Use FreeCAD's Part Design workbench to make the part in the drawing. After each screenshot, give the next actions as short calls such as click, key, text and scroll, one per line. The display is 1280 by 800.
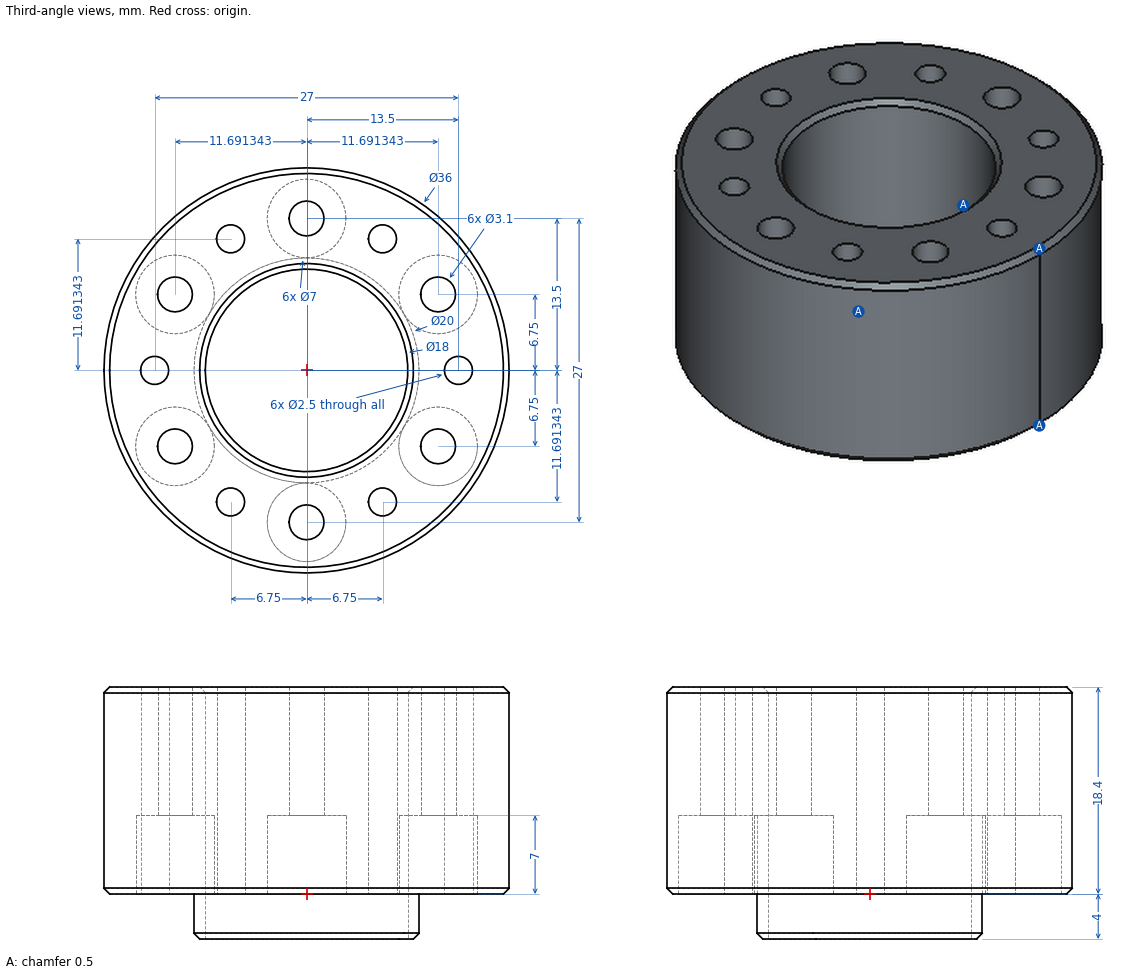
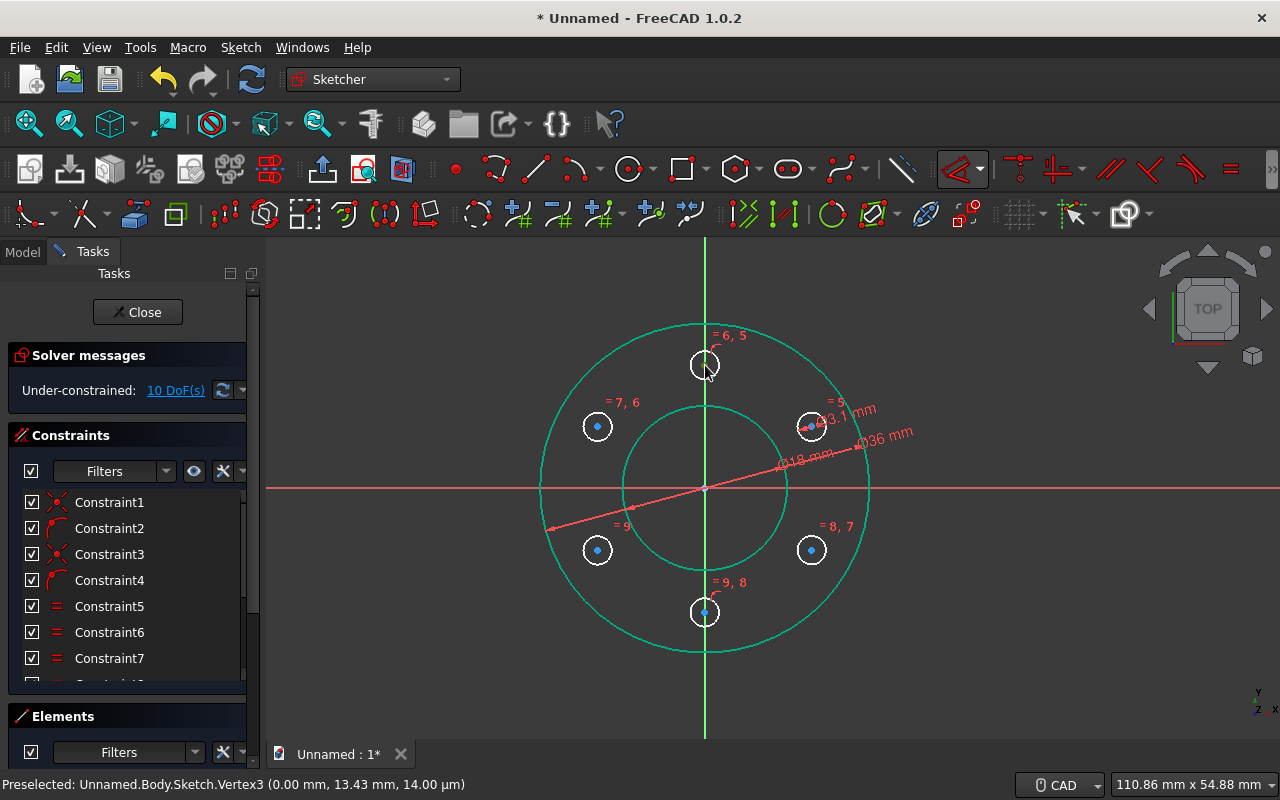
click(705, 612)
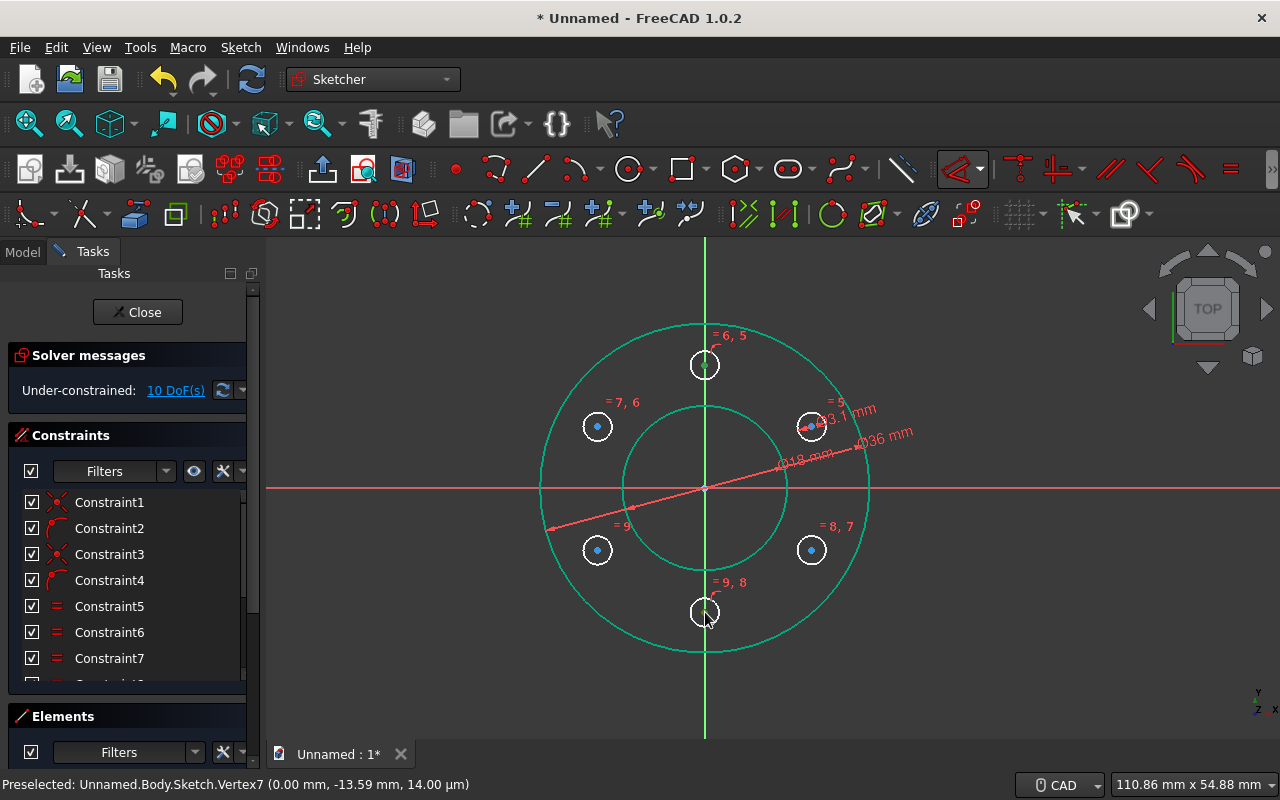
click(982, 170)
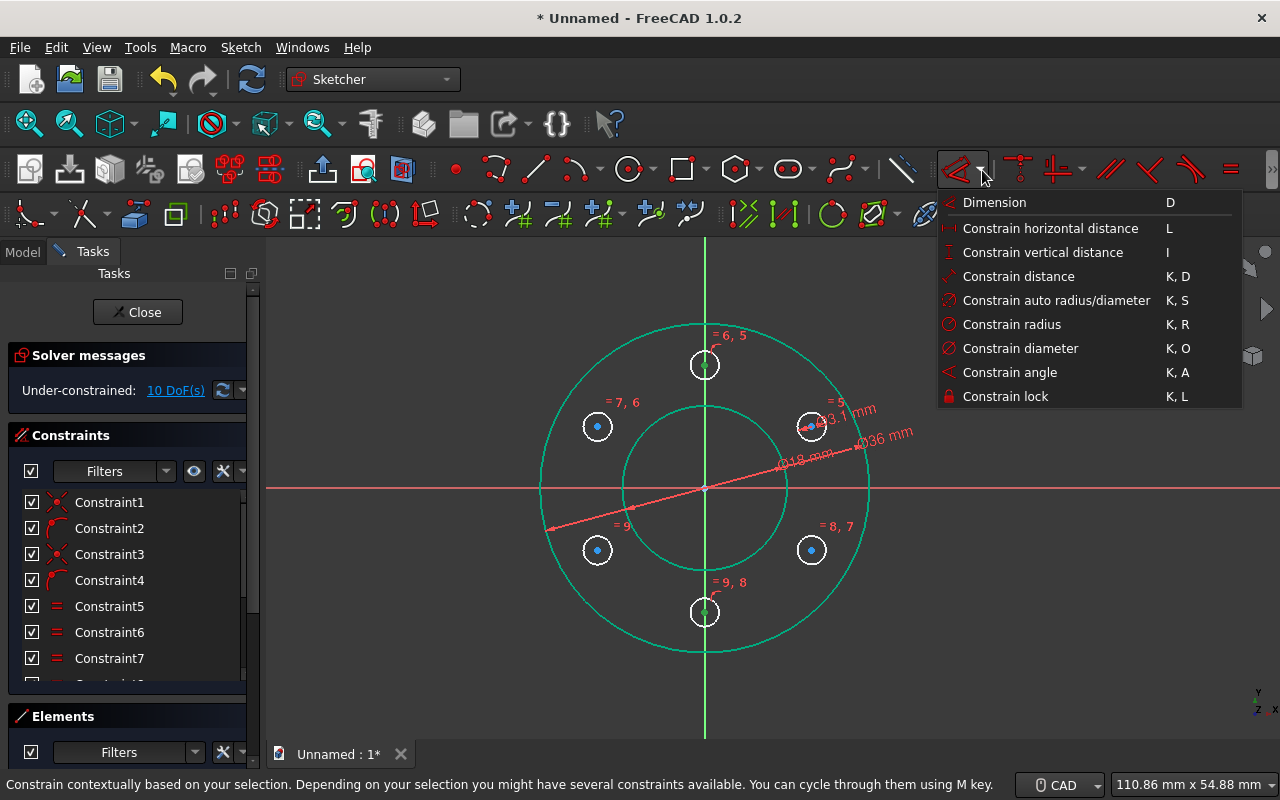
click(1090, 252)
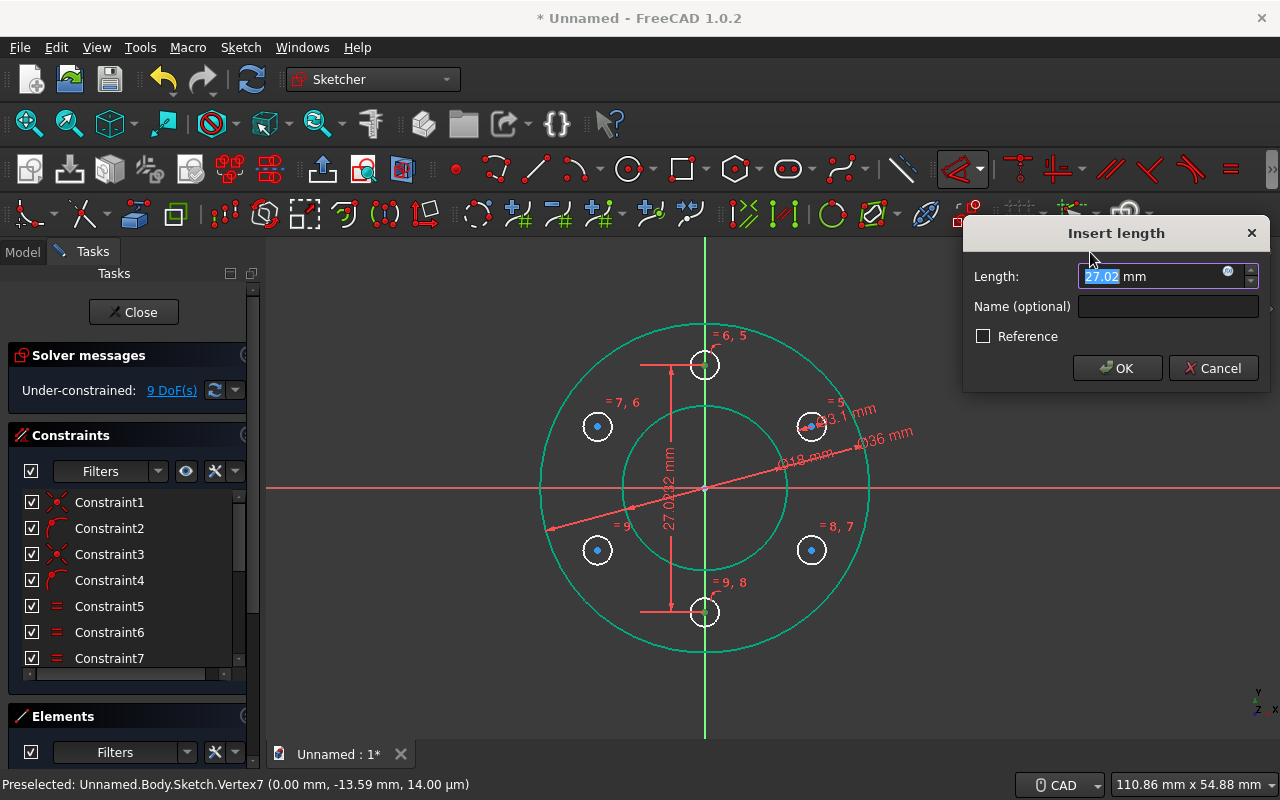
text(27)
key(Return)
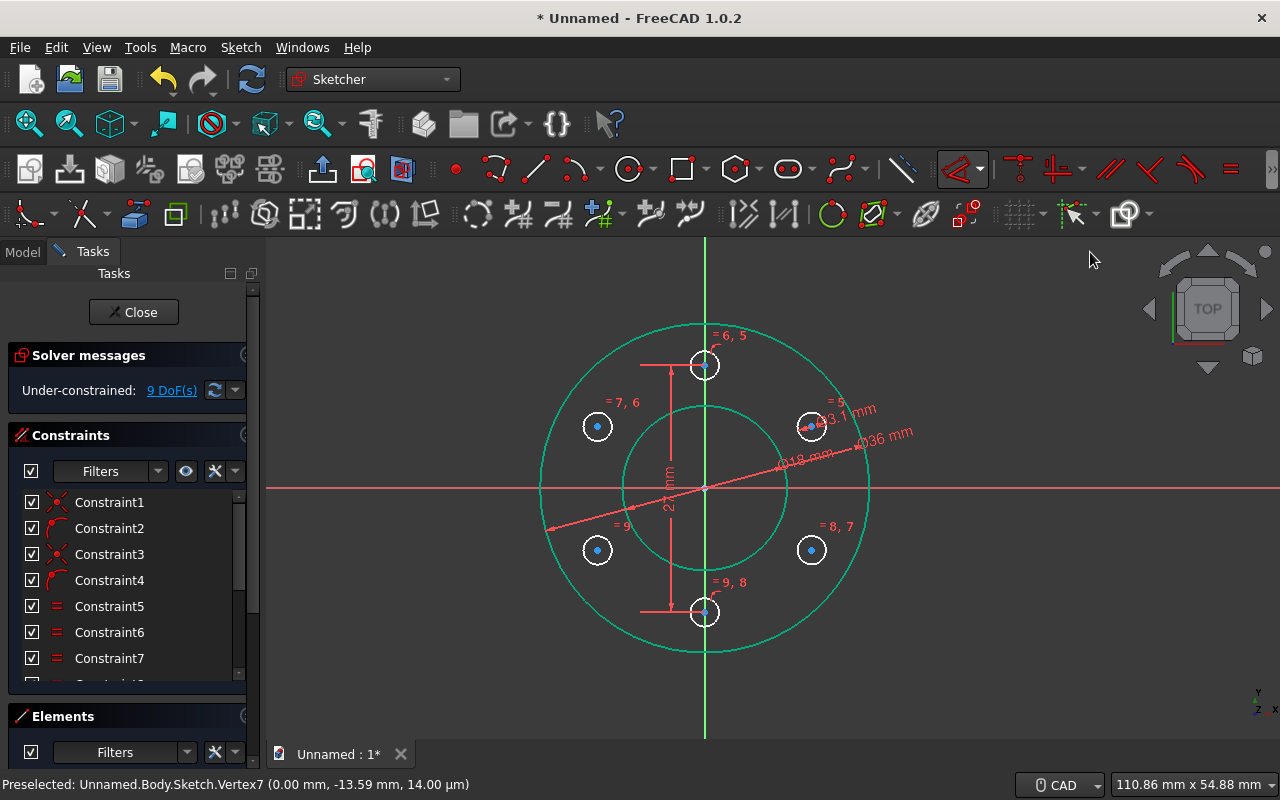
click(812, 427)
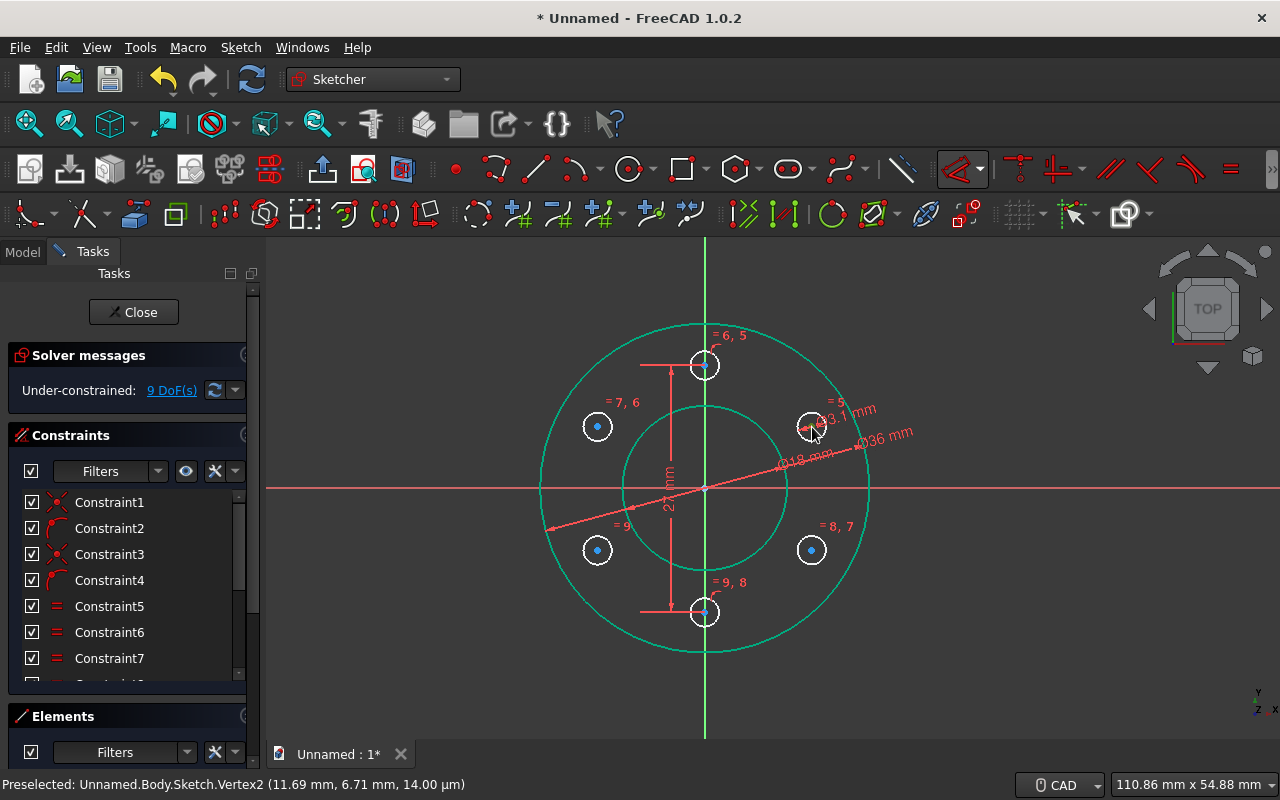
click(982, 170)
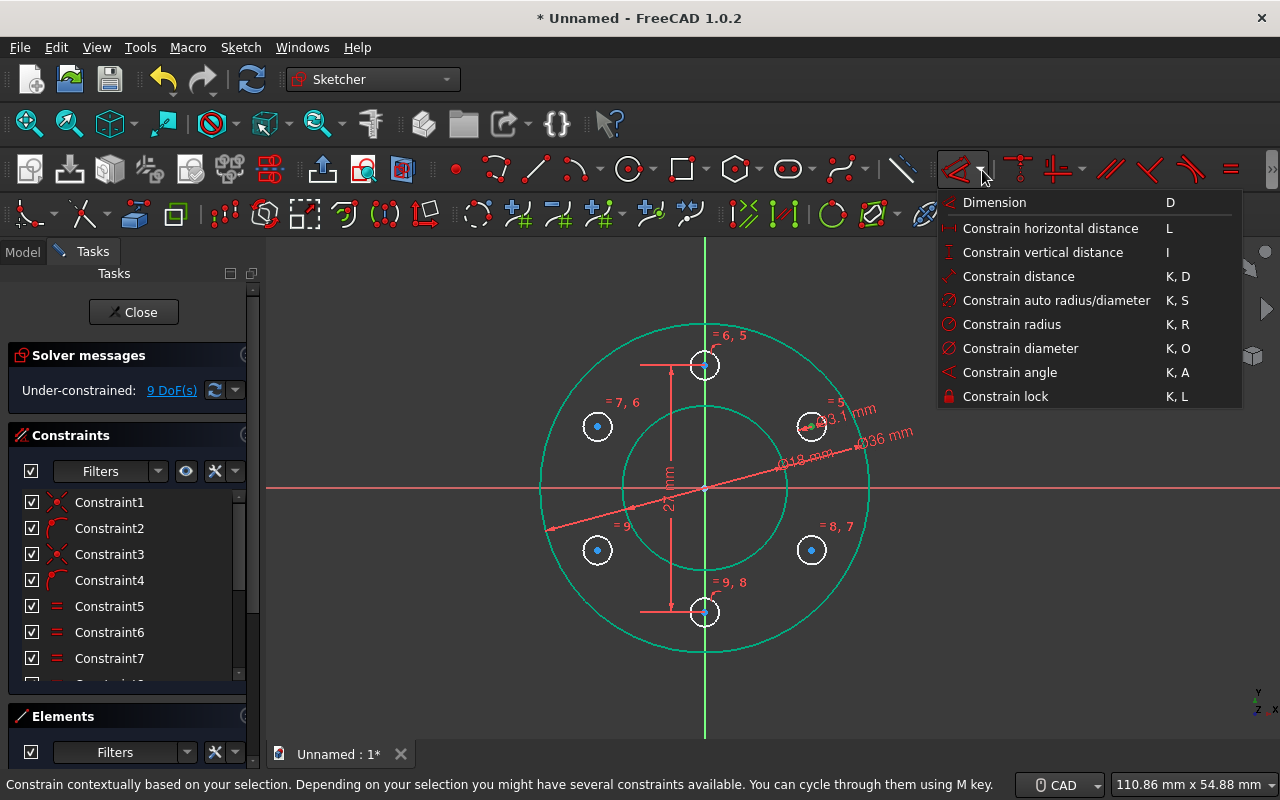
click(1090, 252)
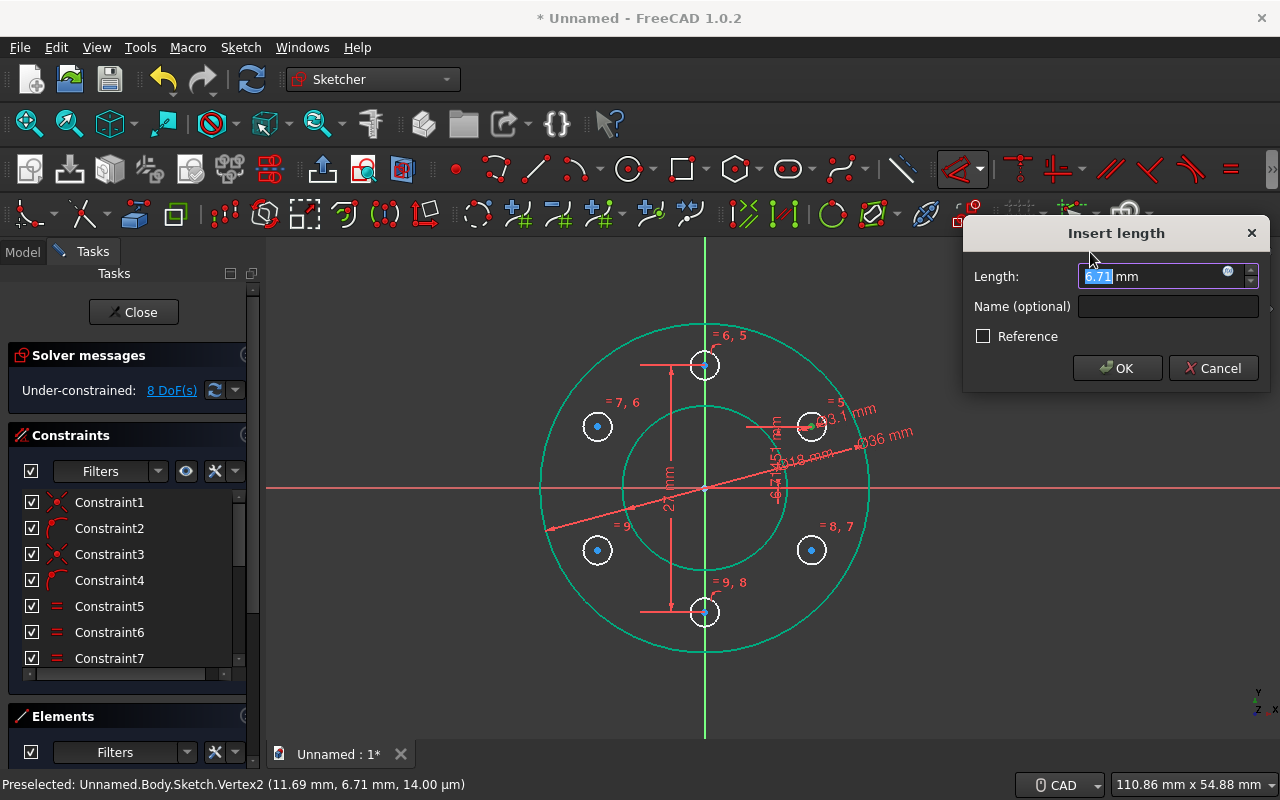
text(6.75)
key(Return)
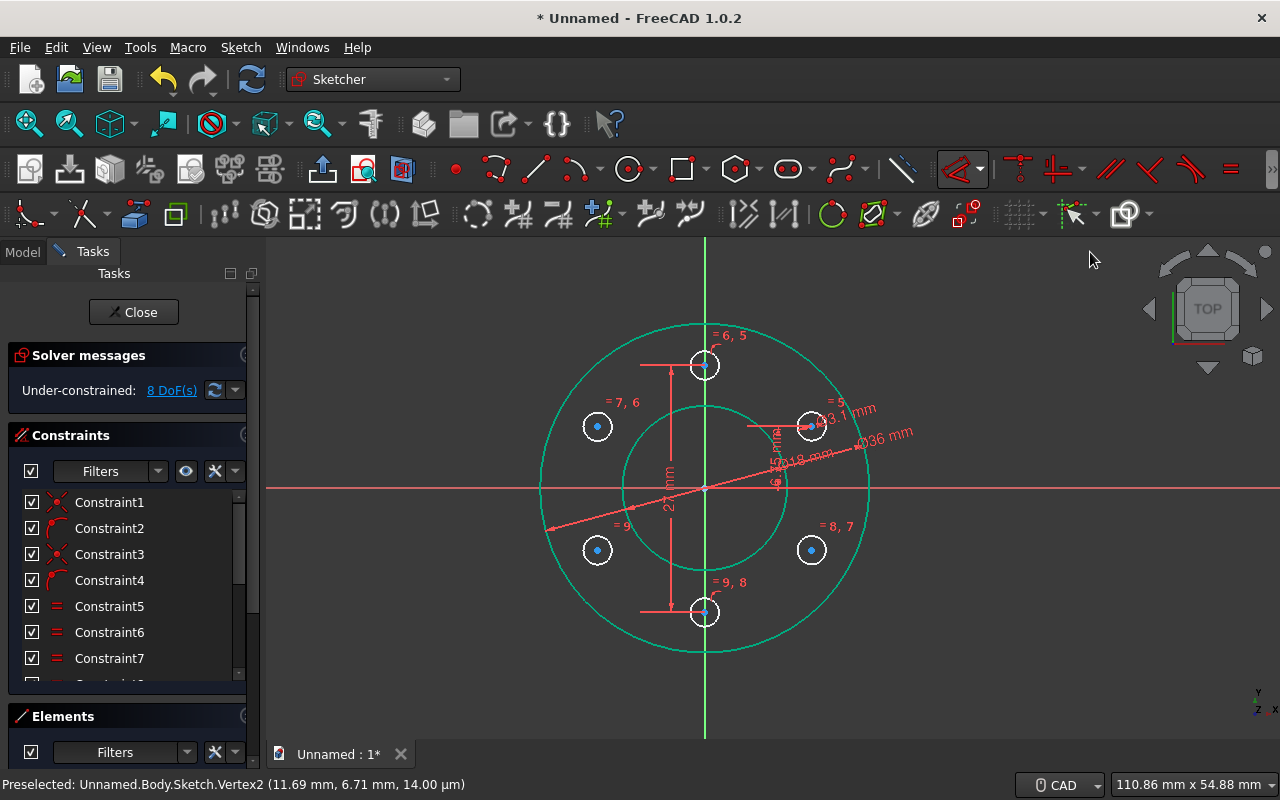
click(705, 365)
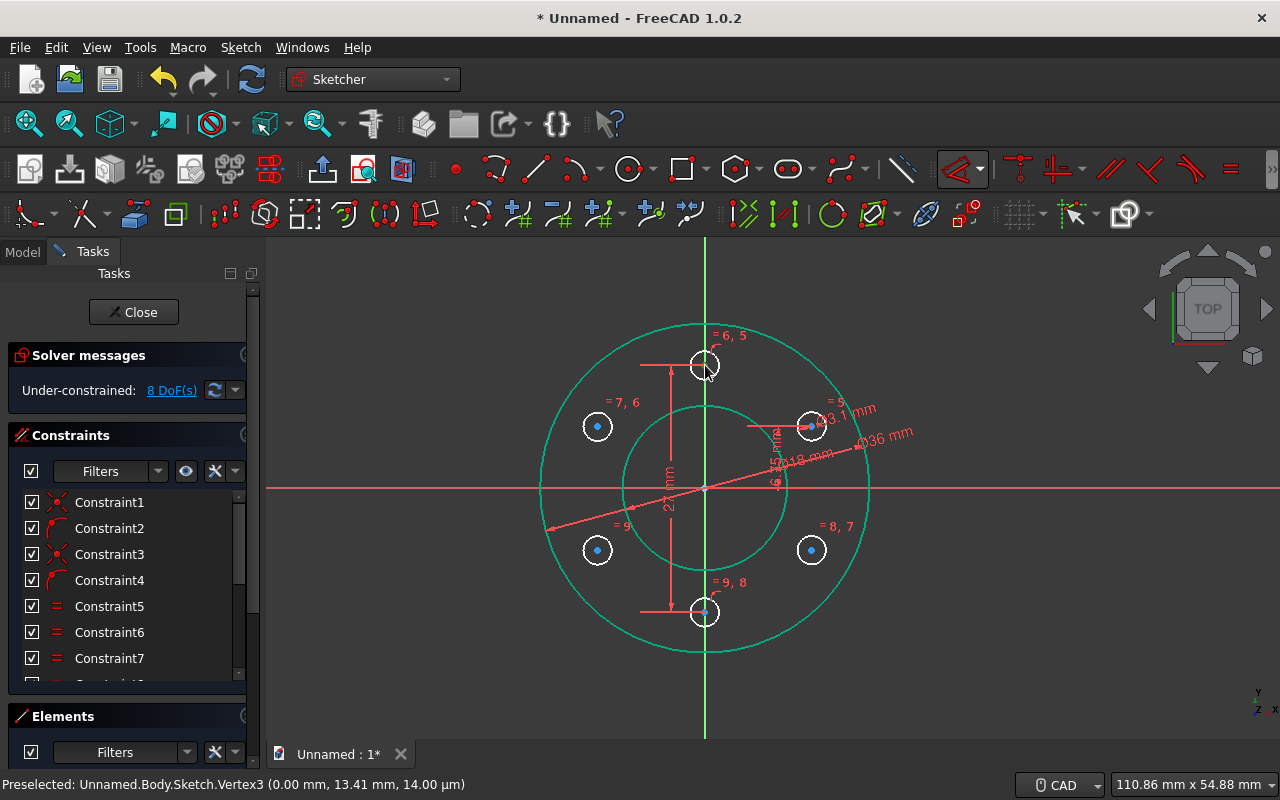
key(i)